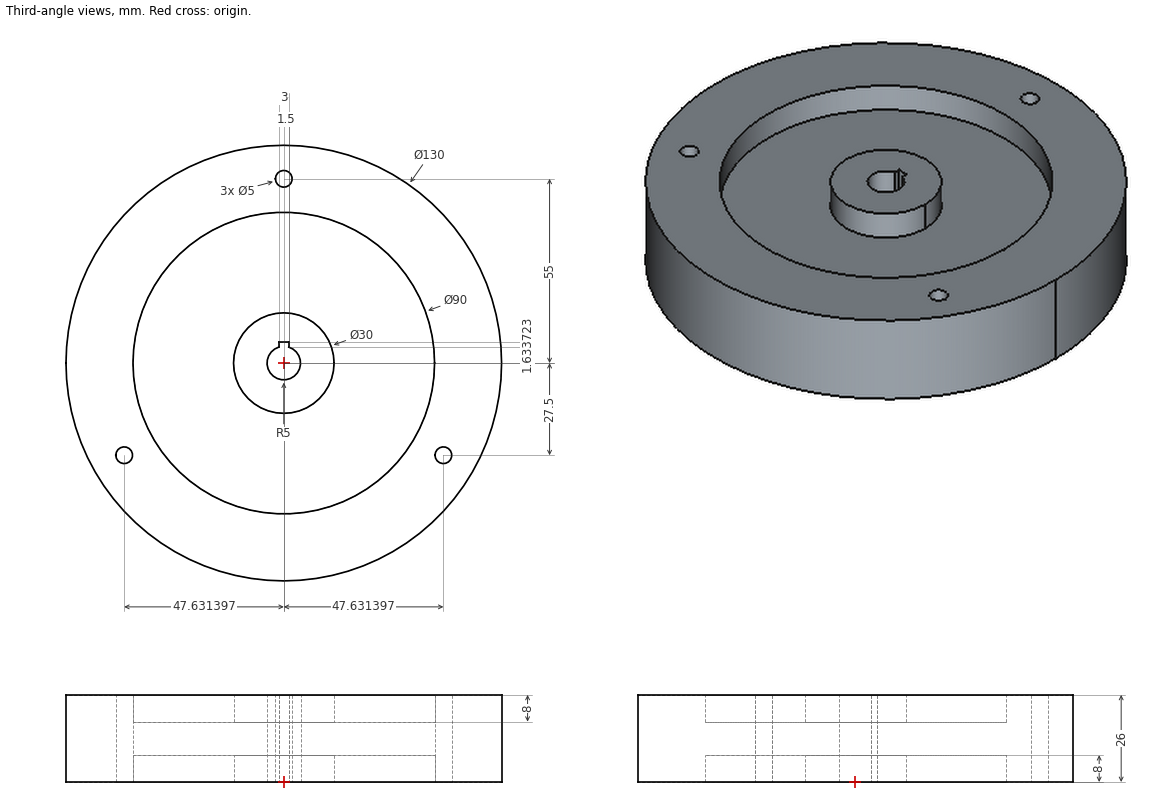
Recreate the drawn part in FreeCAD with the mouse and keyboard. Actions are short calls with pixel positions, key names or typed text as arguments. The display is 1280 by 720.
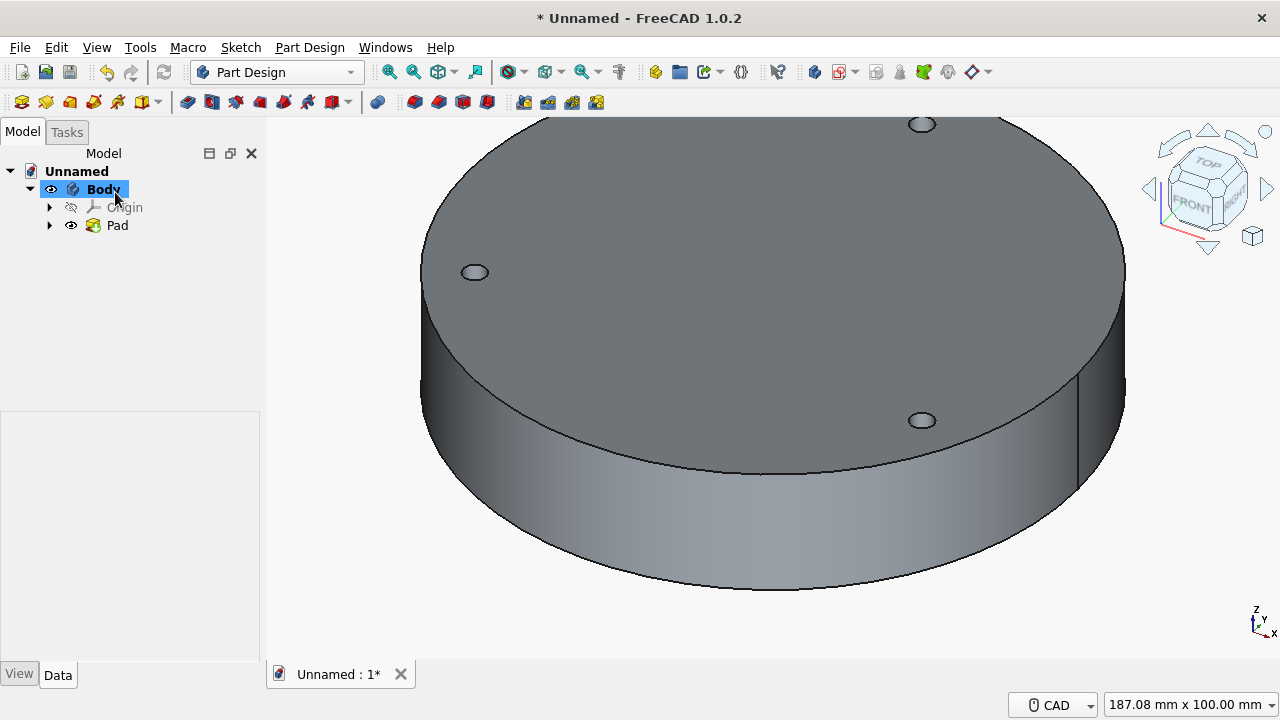
click(390, 72)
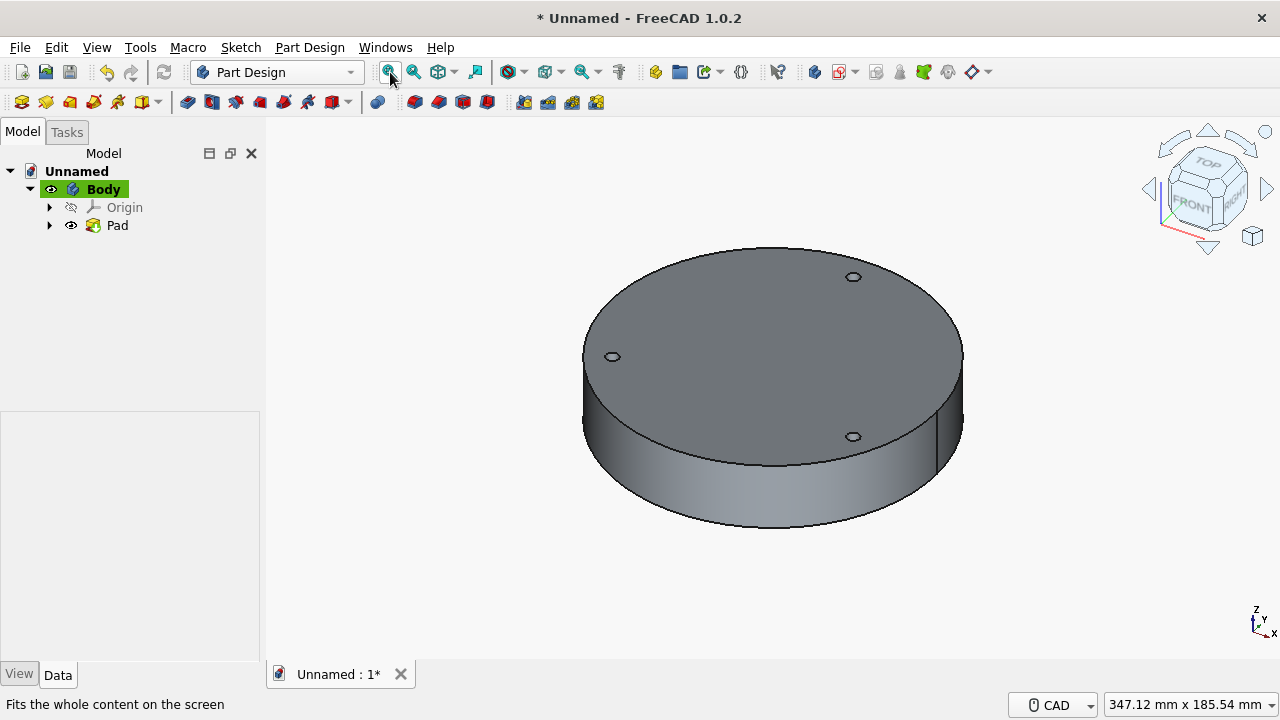
click(773, 356)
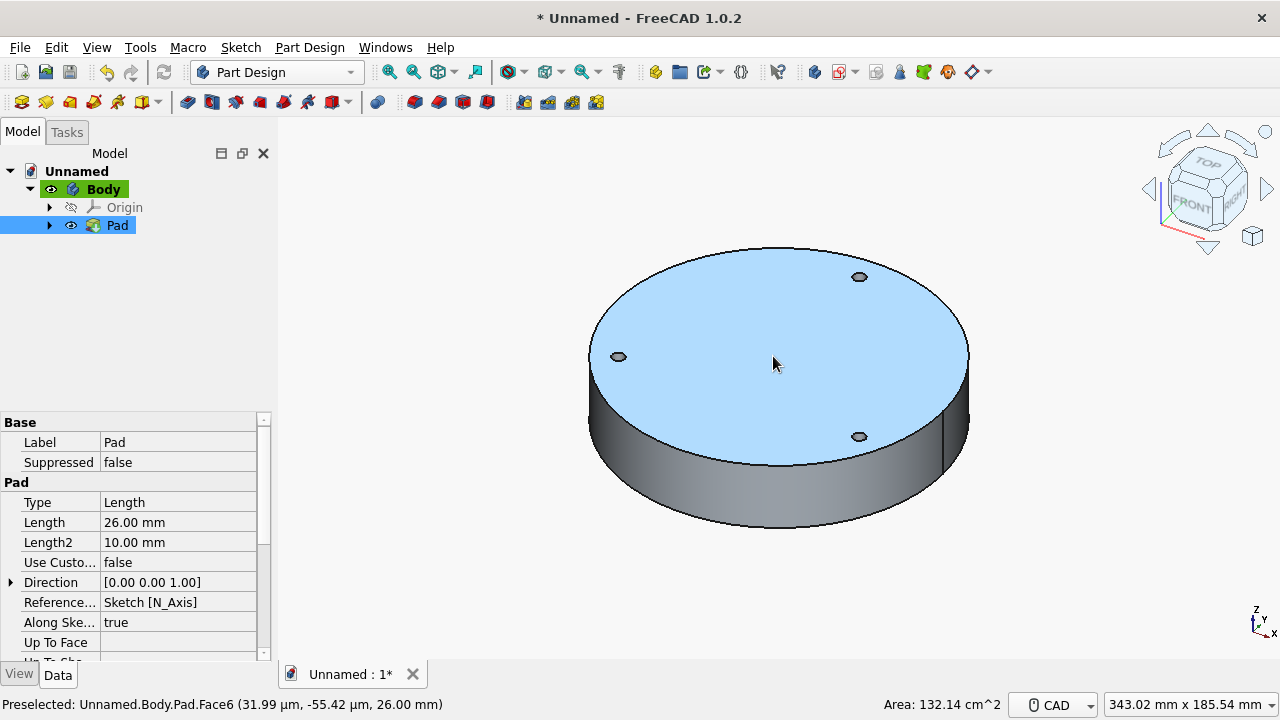
click(840, 72)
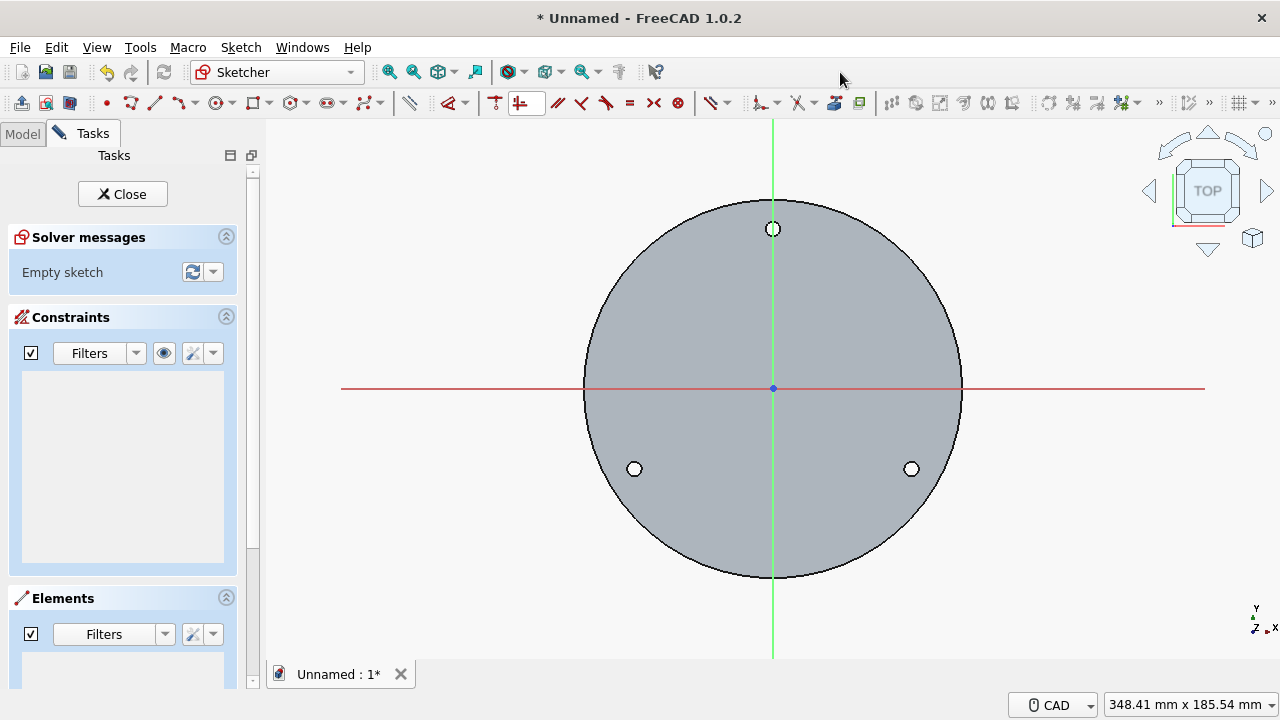
scroll(780, 387, up, 12)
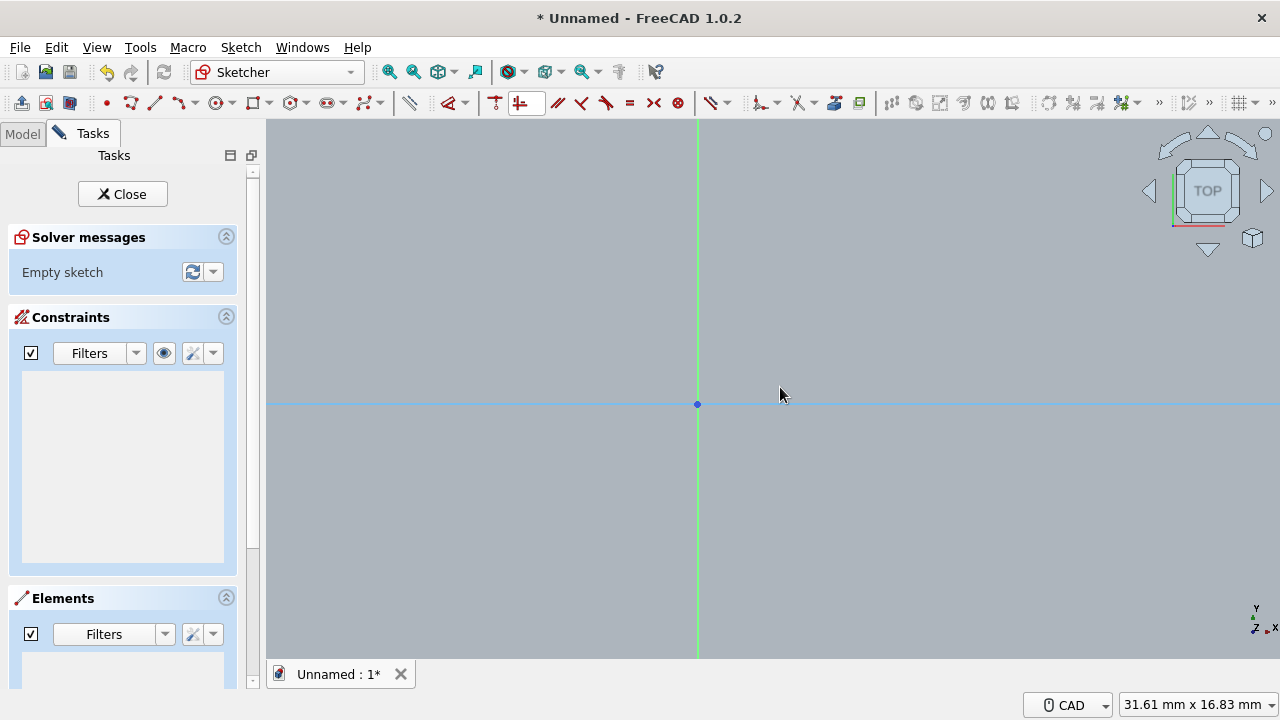
key(g)
key(m)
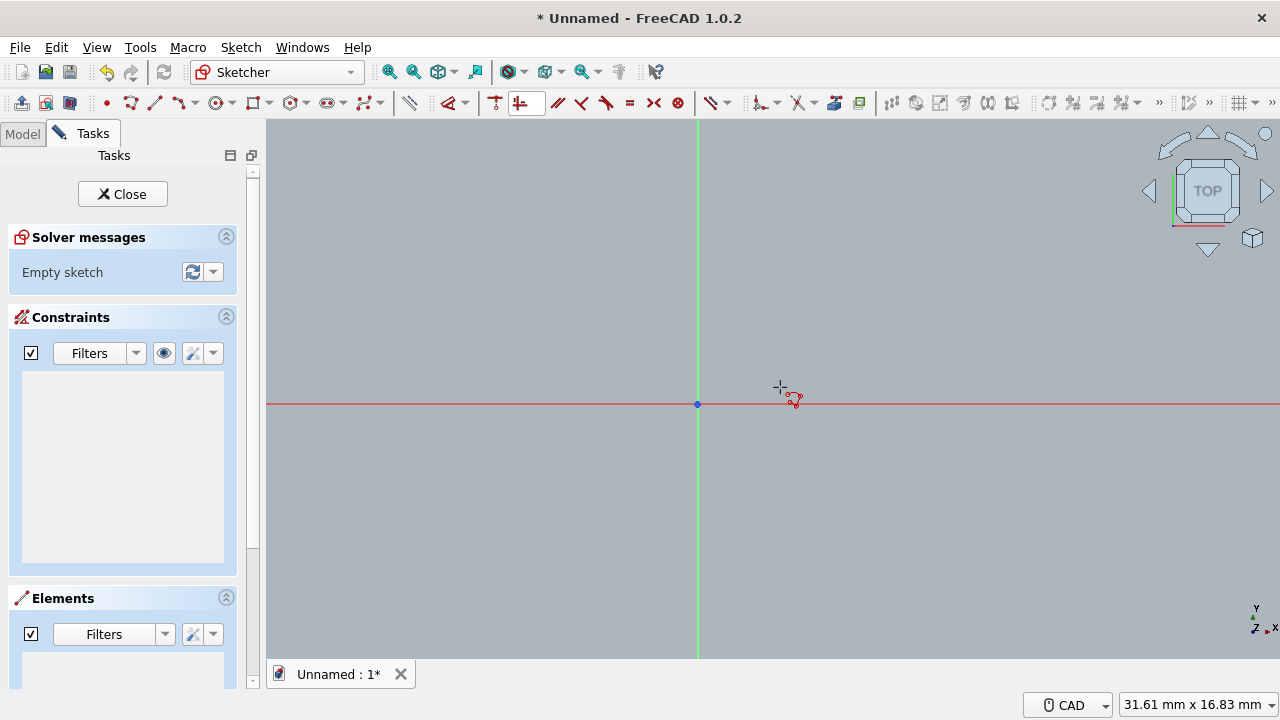
click(746, 251)
click(746, 199)
click(650, 199)
click(650, 251)
right_click(650, 251)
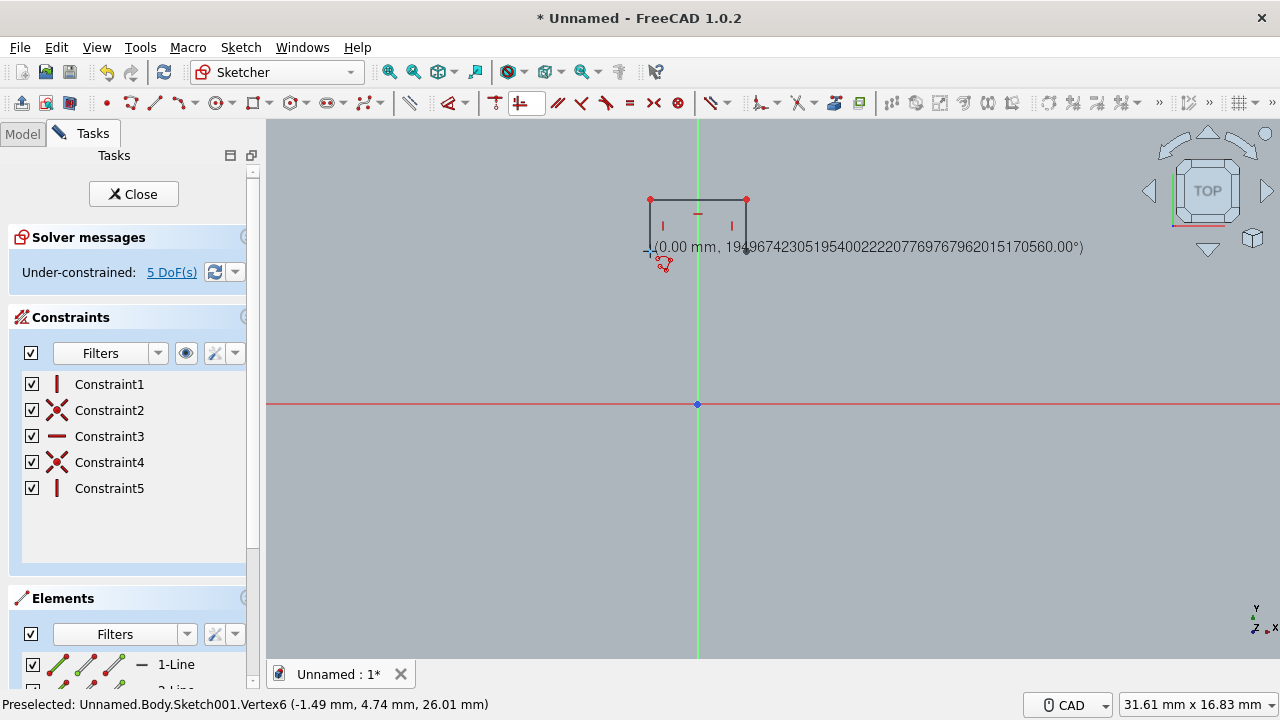
click(180, 104)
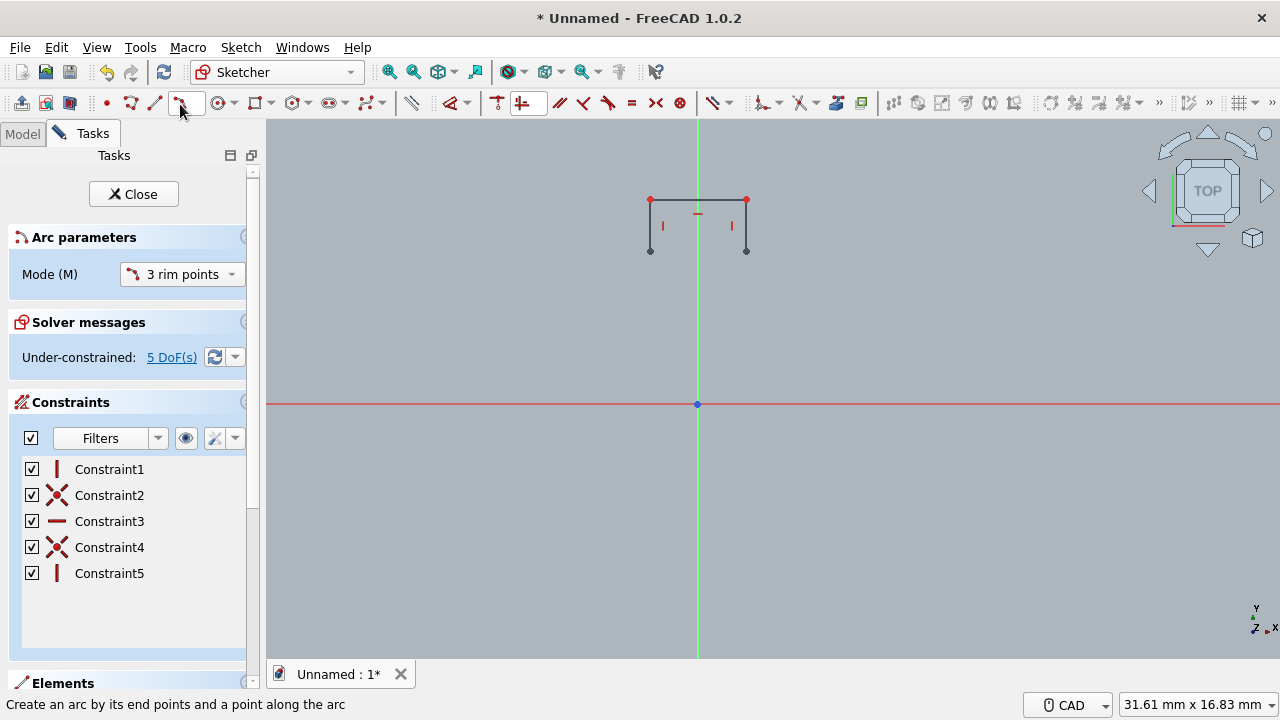
click(650, 252)
click(746, 252)
click(612, 539)
key(Escape)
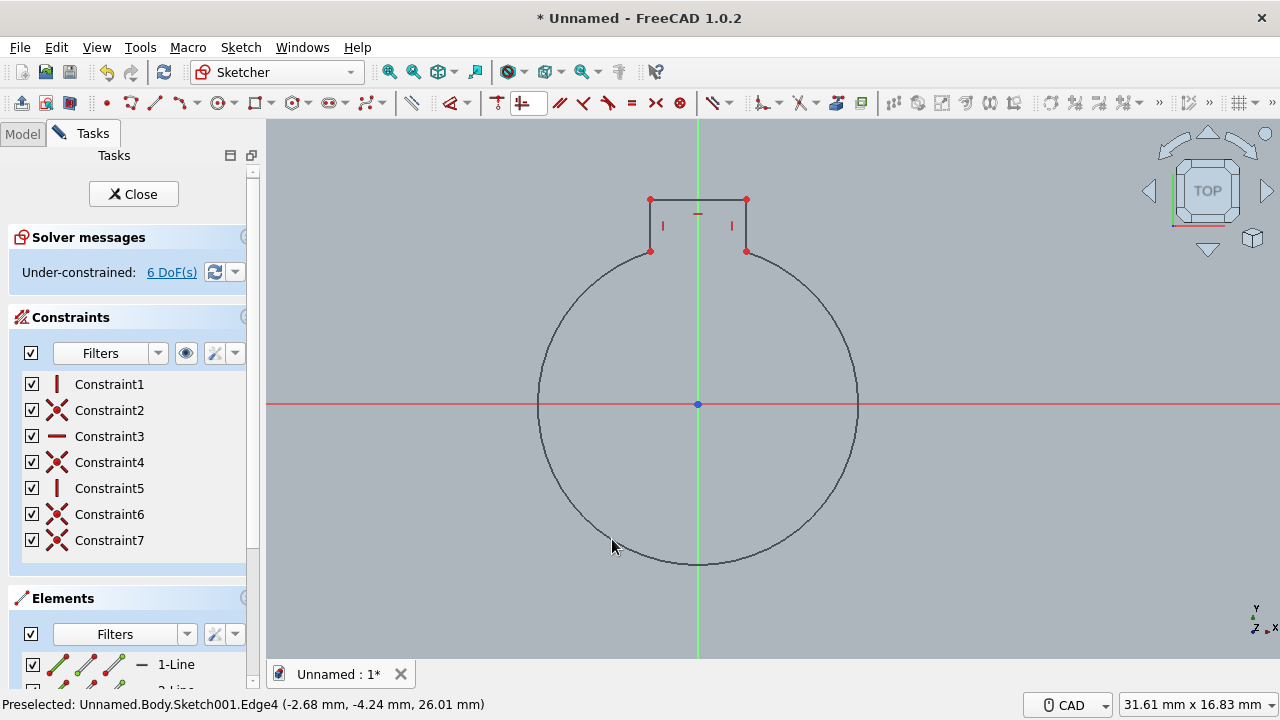
drag(688, 394, 708, 415)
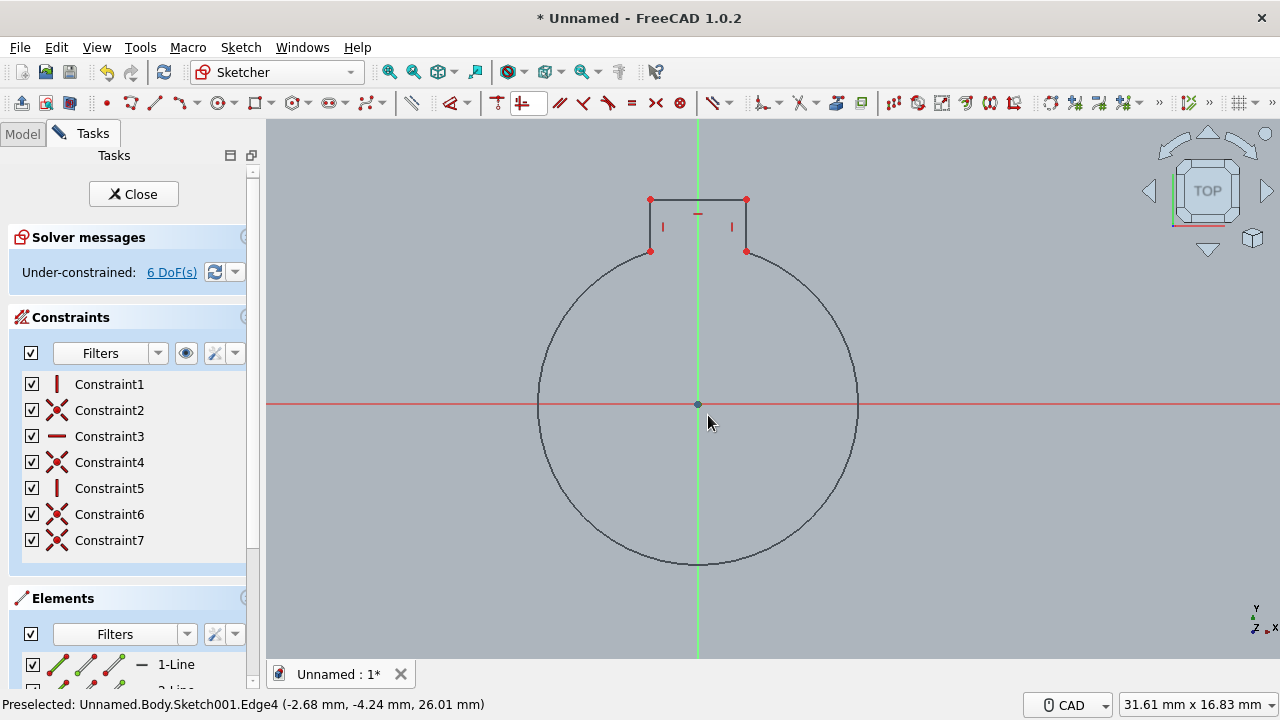
click(498, 104)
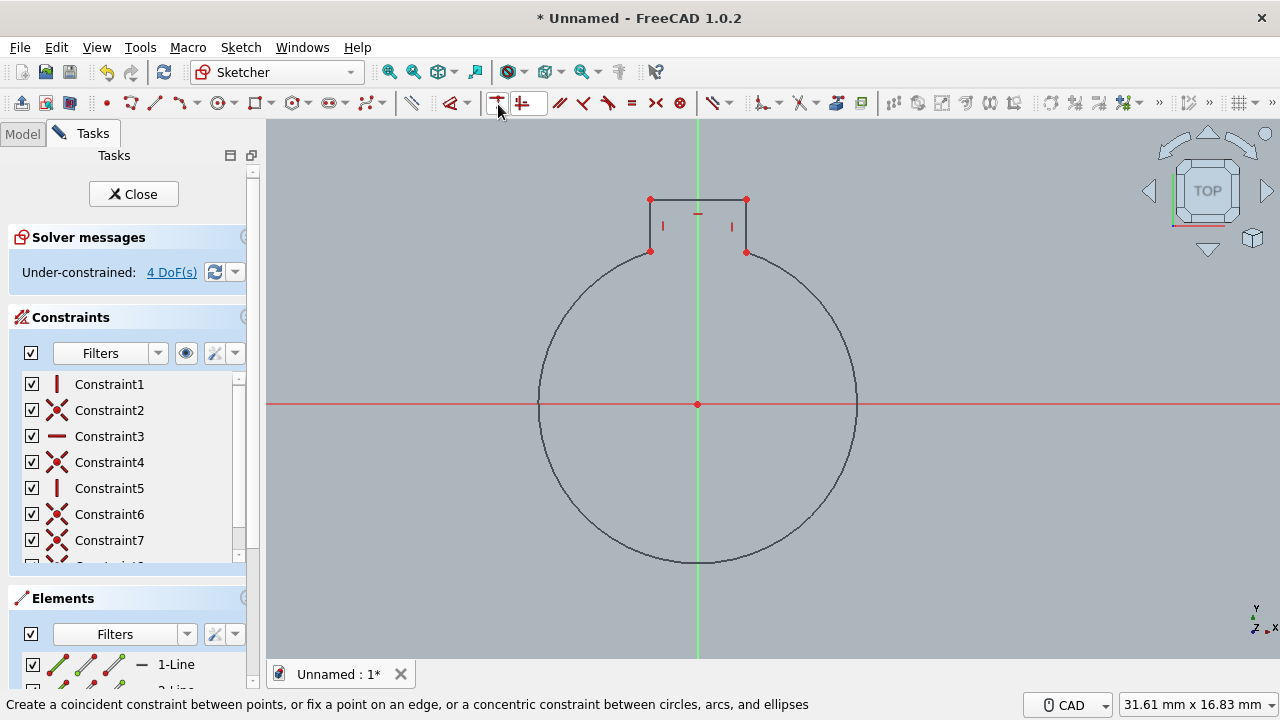
key(d)